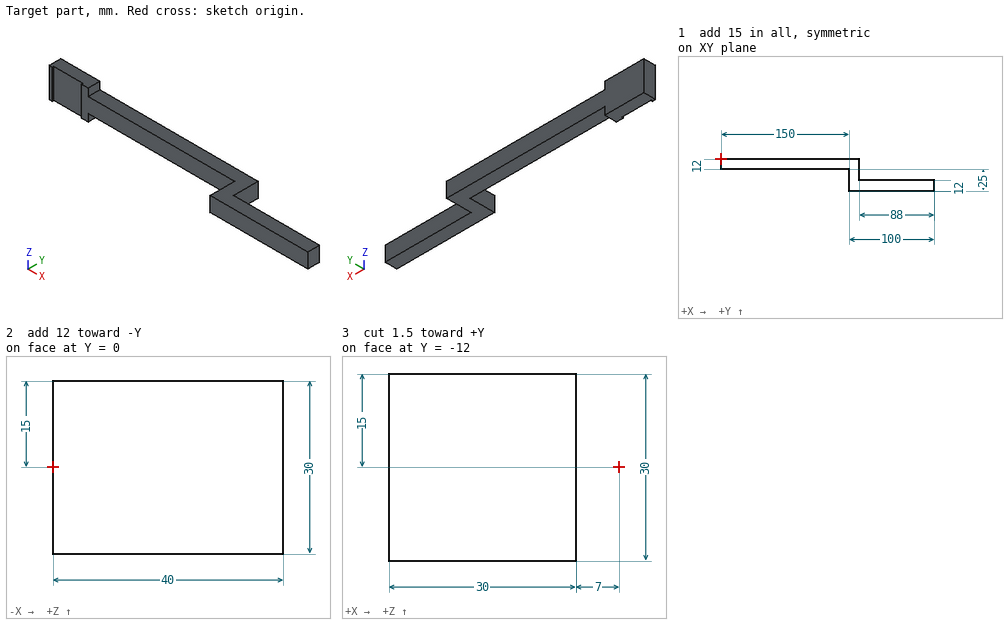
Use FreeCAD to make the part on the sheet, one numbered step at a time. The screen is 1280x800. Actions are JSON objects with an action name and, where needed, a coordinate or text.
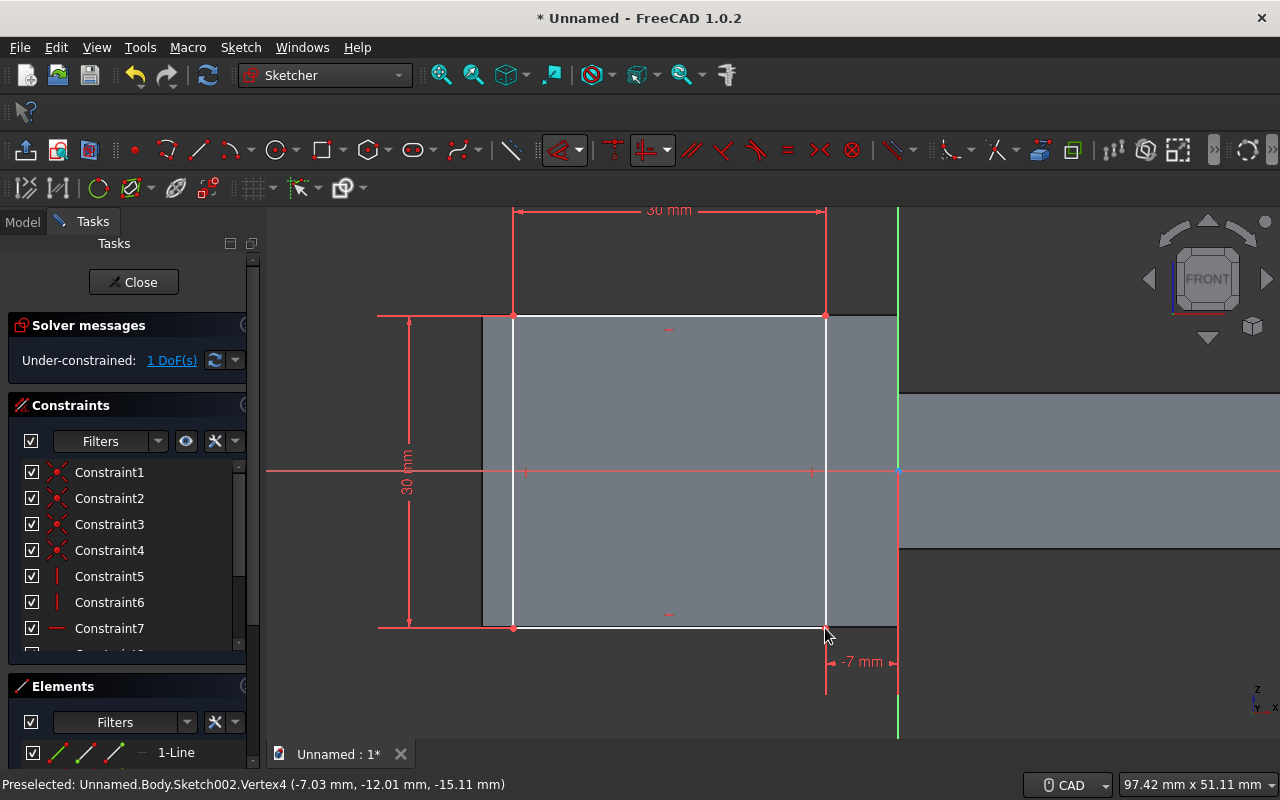
{"action": "left_click", "coordinate": [513, 316]}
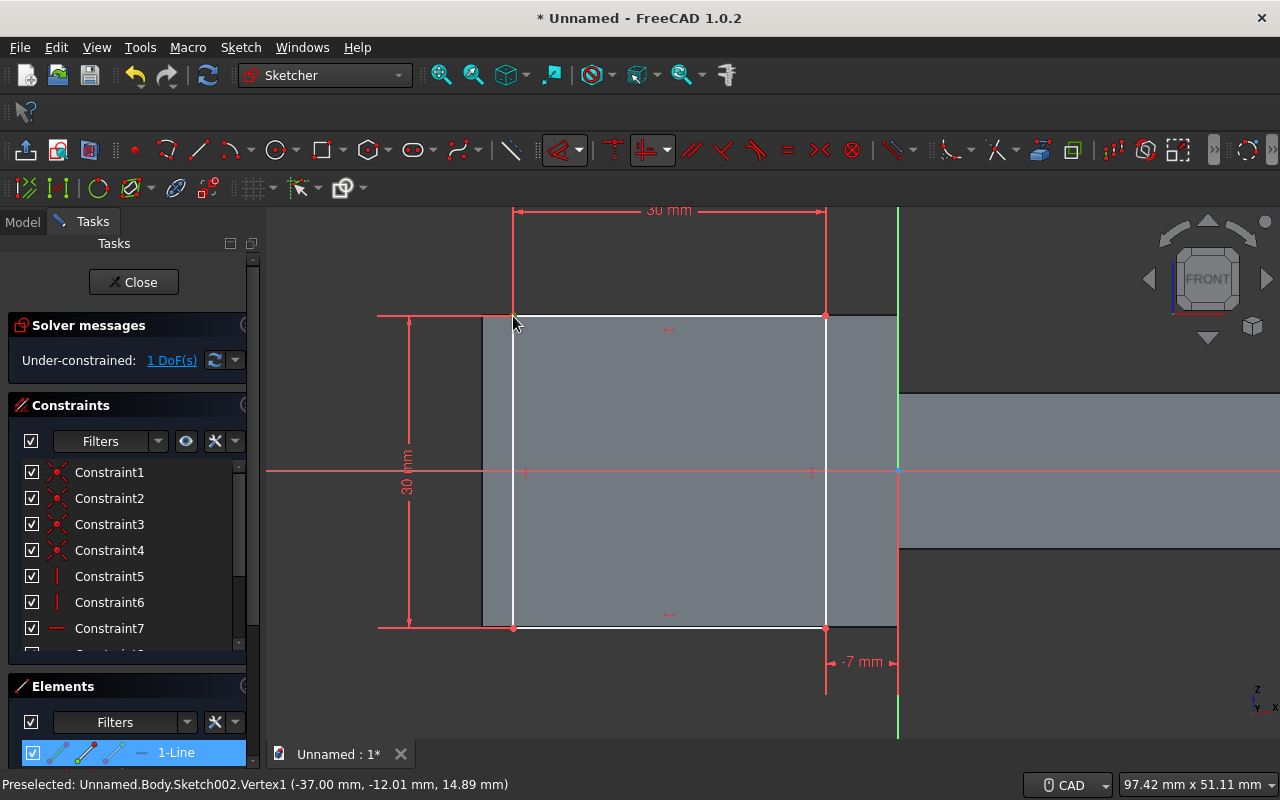
{"action": "left_click", "coordinate": [582, 150]}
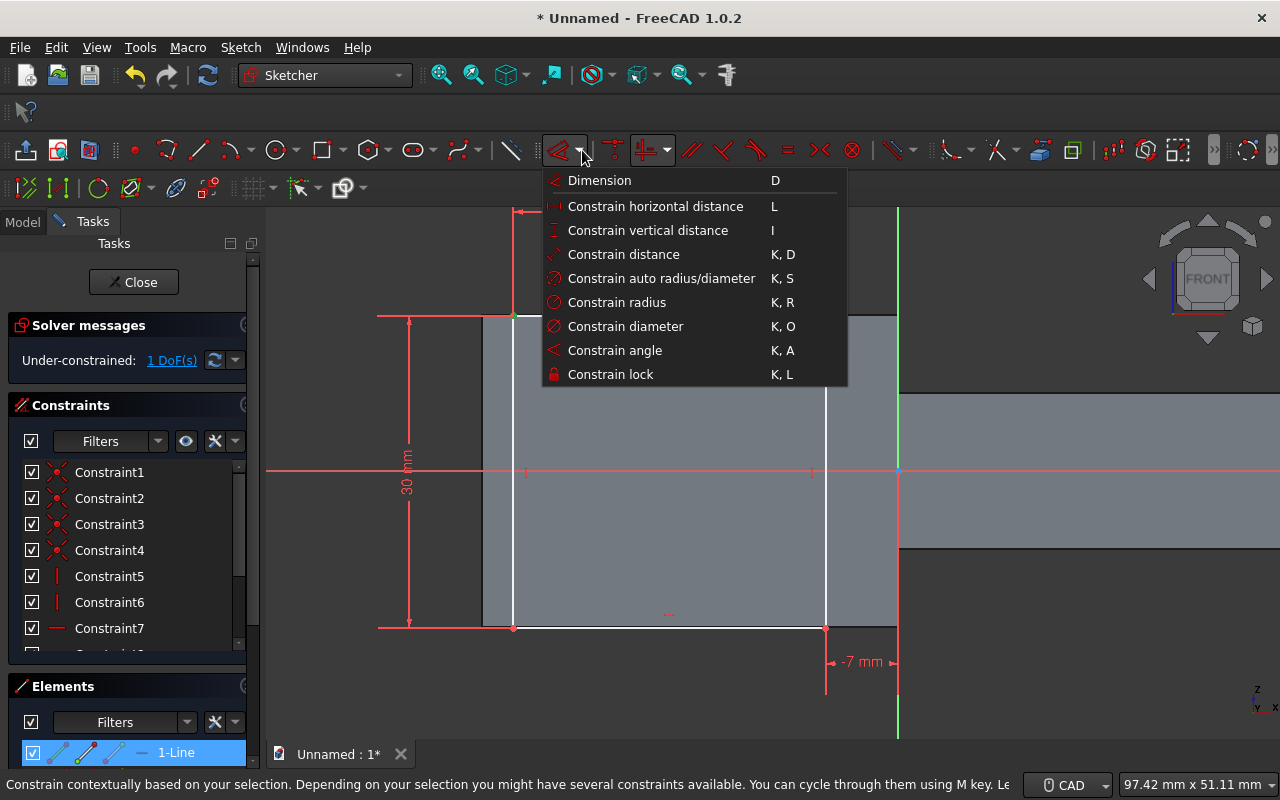
{"action": "left_click", "coordinate": [695, 230]}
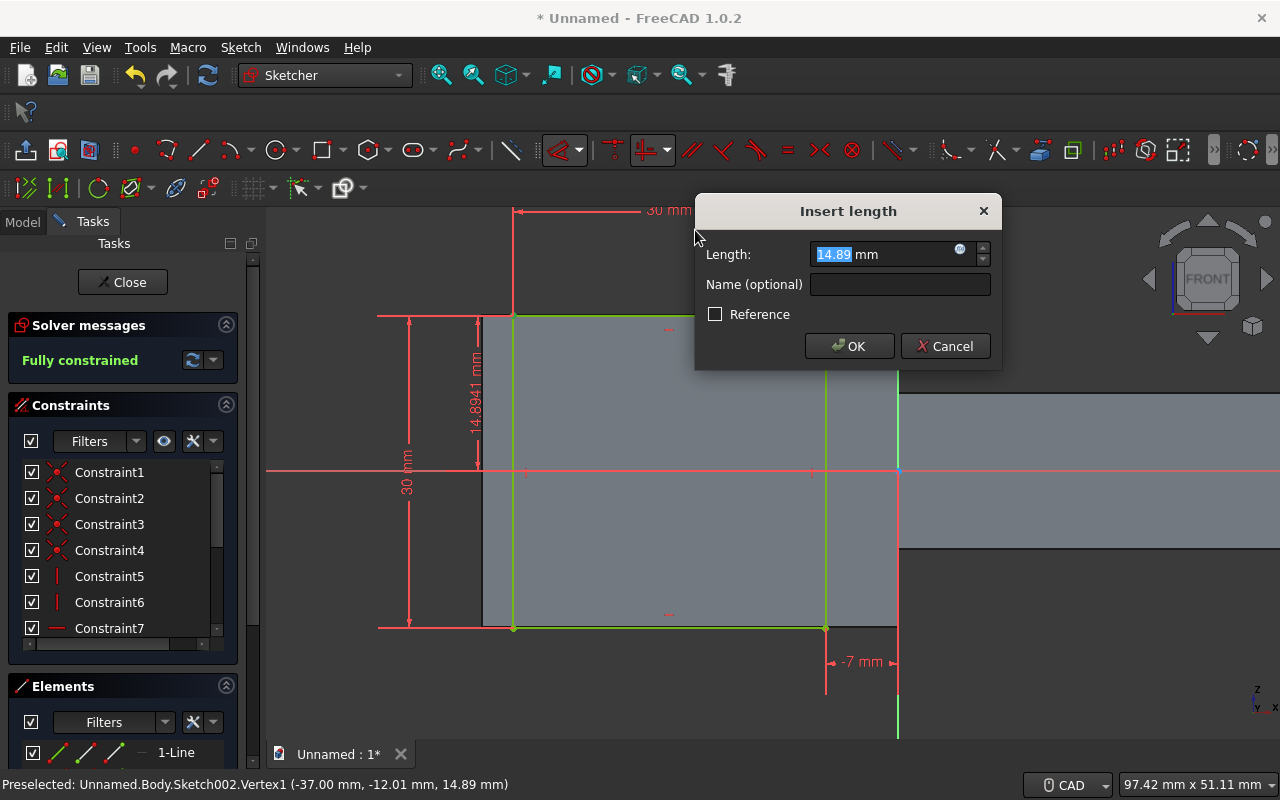
{"action": "type", "text": "15"}
{"action": "key", "text": "Return"}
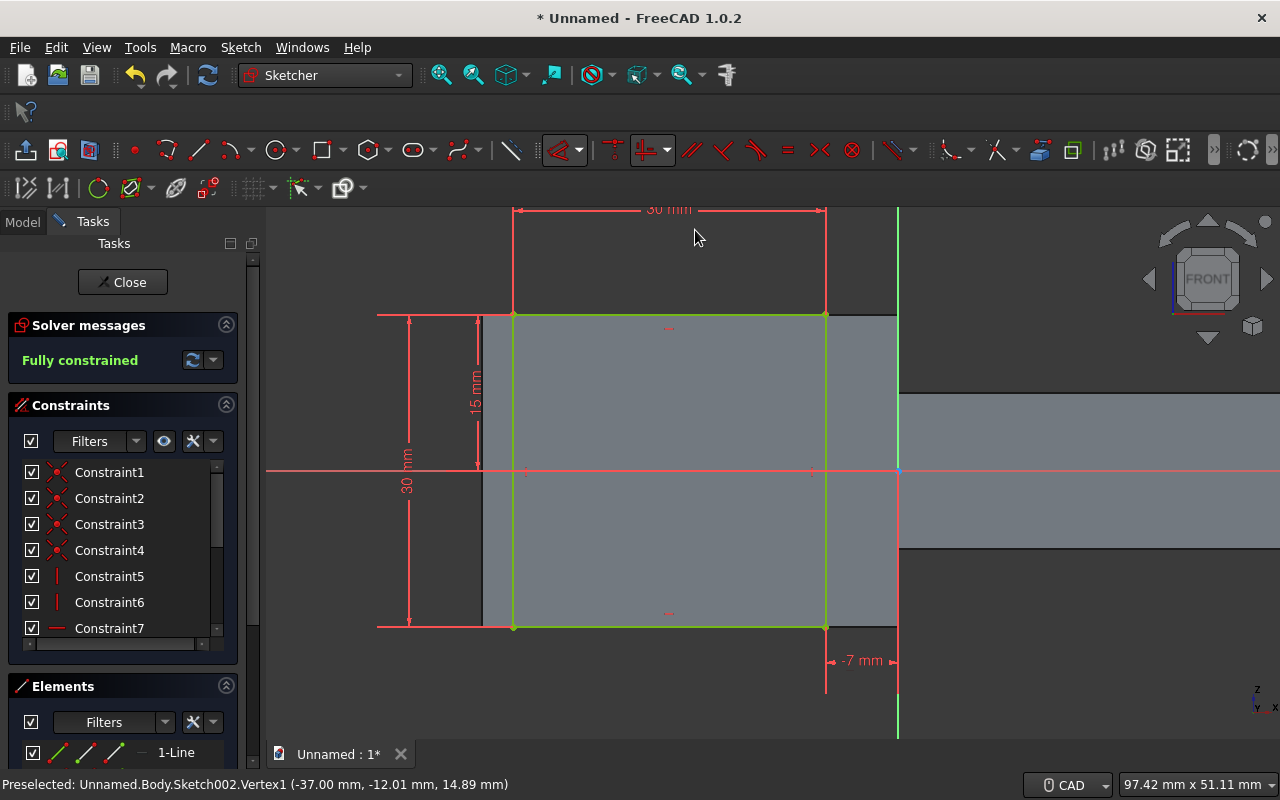
{"action": "left_click", "coordinate": [123, 282]}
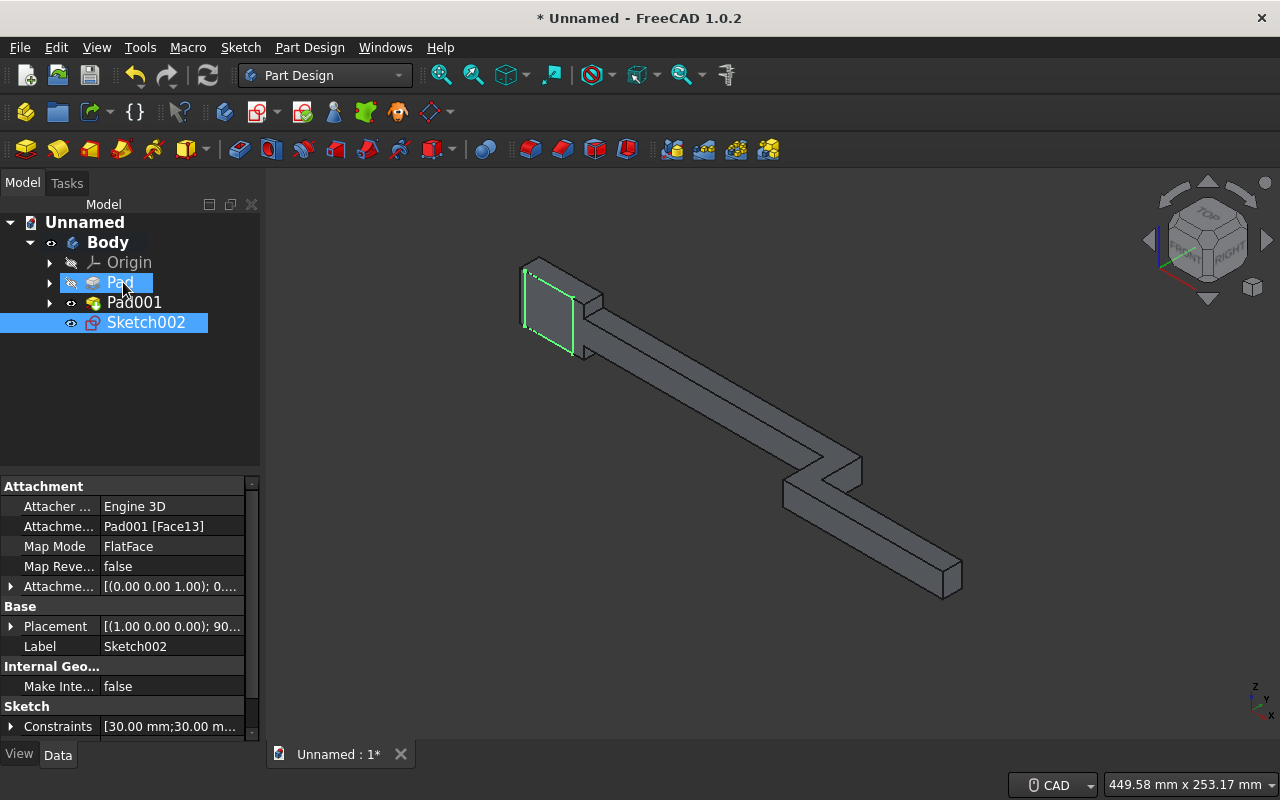
{"action": "left_click", "coordinate": [240, 150]}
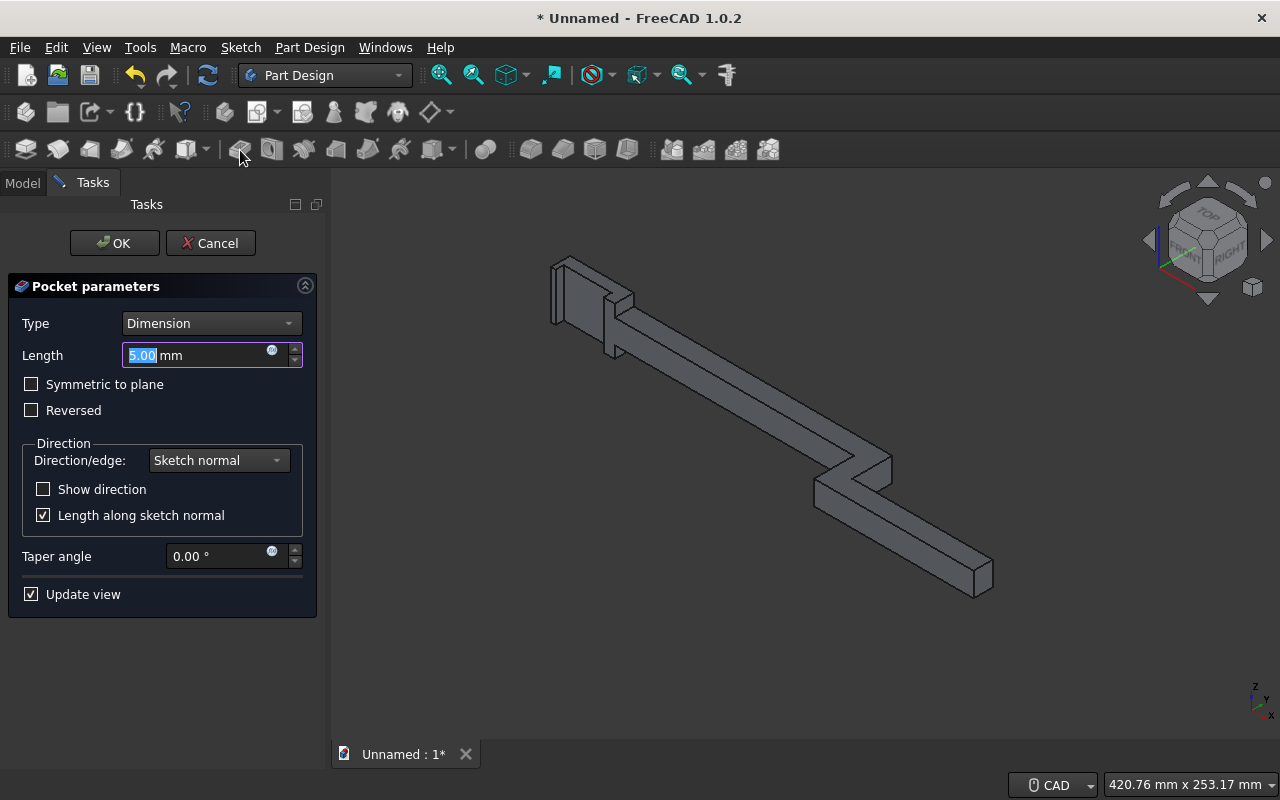
{"action": "type", "text": "1.5"}
{"action": "key", "text": "Tab"}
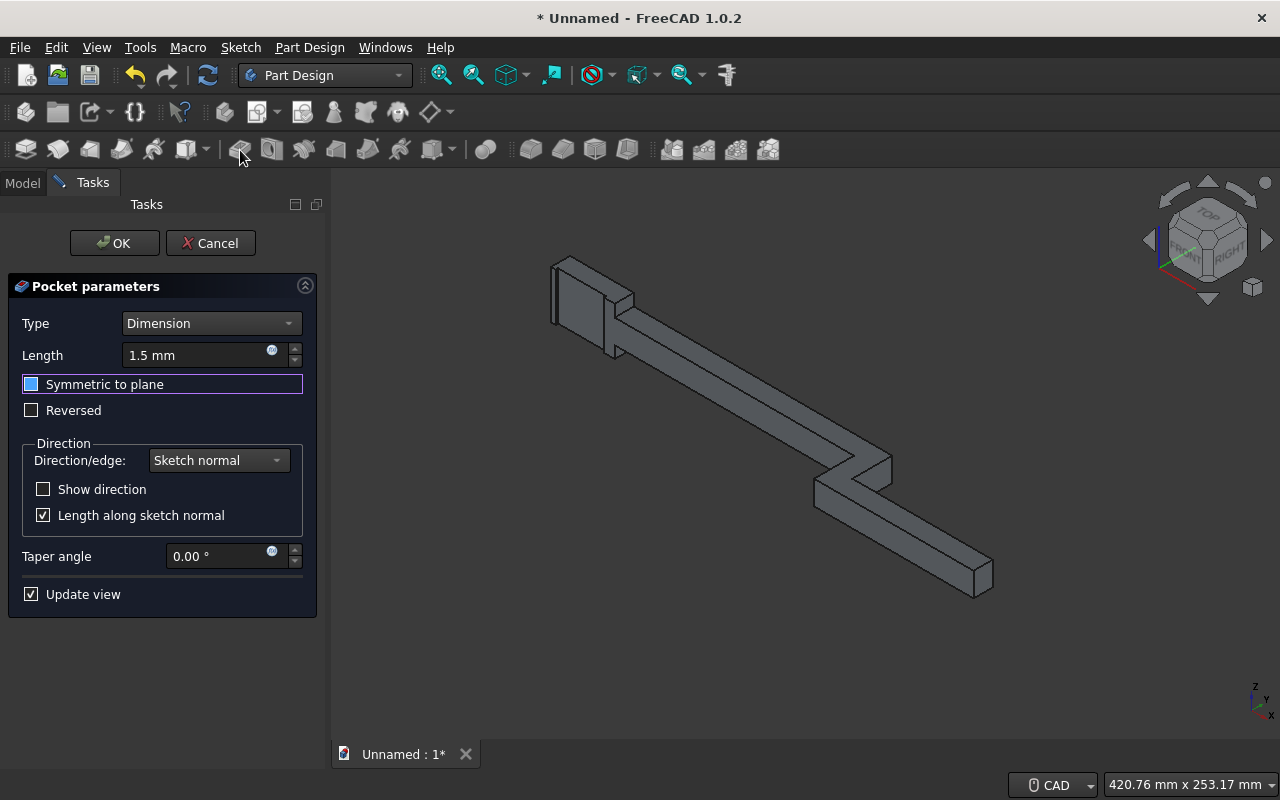
{"action": "left_click", "coordinate": [115, 243]}